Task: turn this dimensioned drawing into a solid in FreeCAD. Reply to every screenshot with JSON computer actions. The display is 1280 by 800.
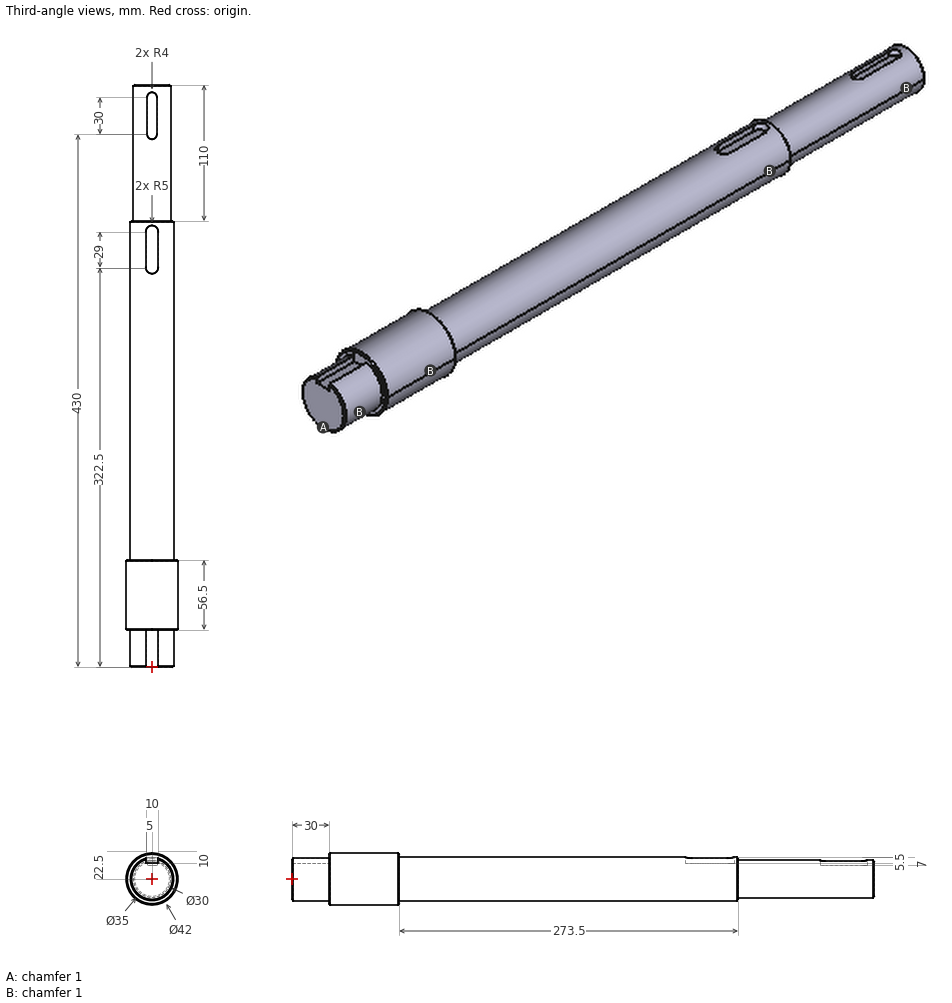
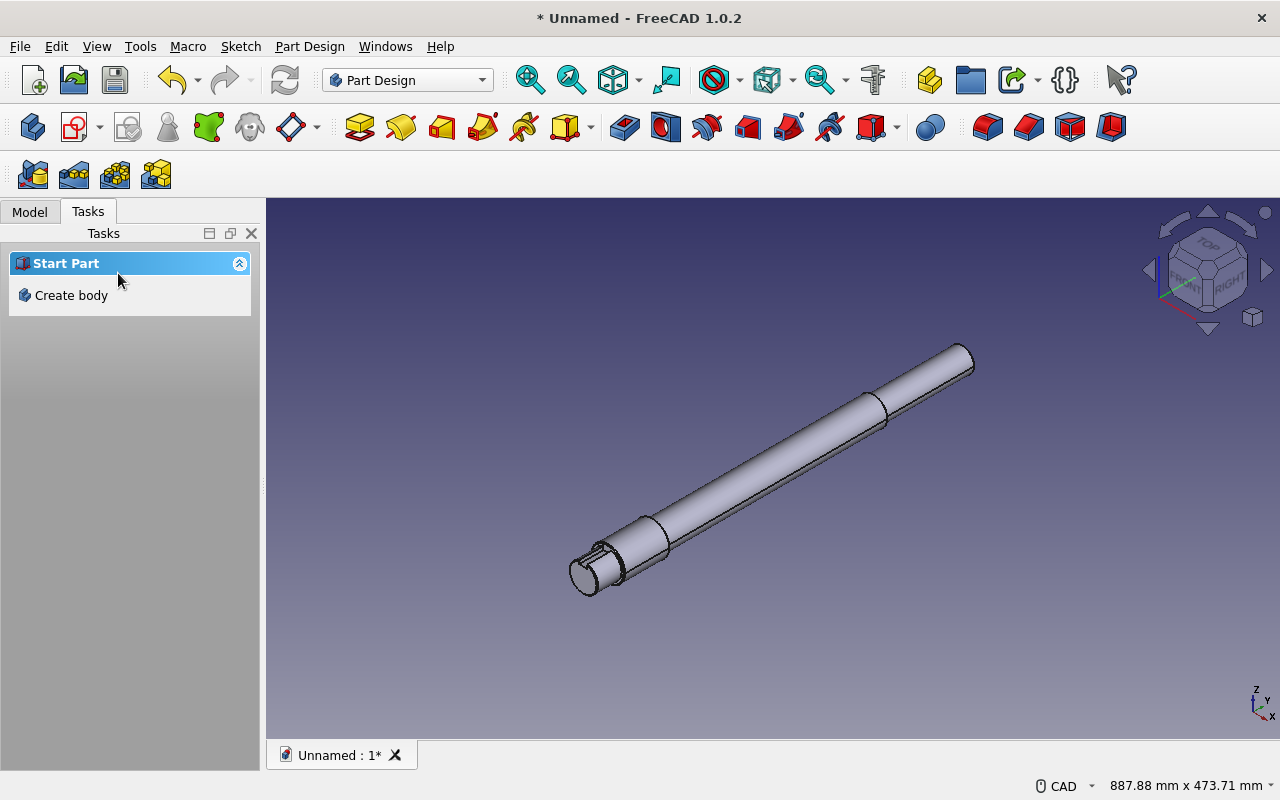
{"action": "left_click", "coordinate": [30, 212]}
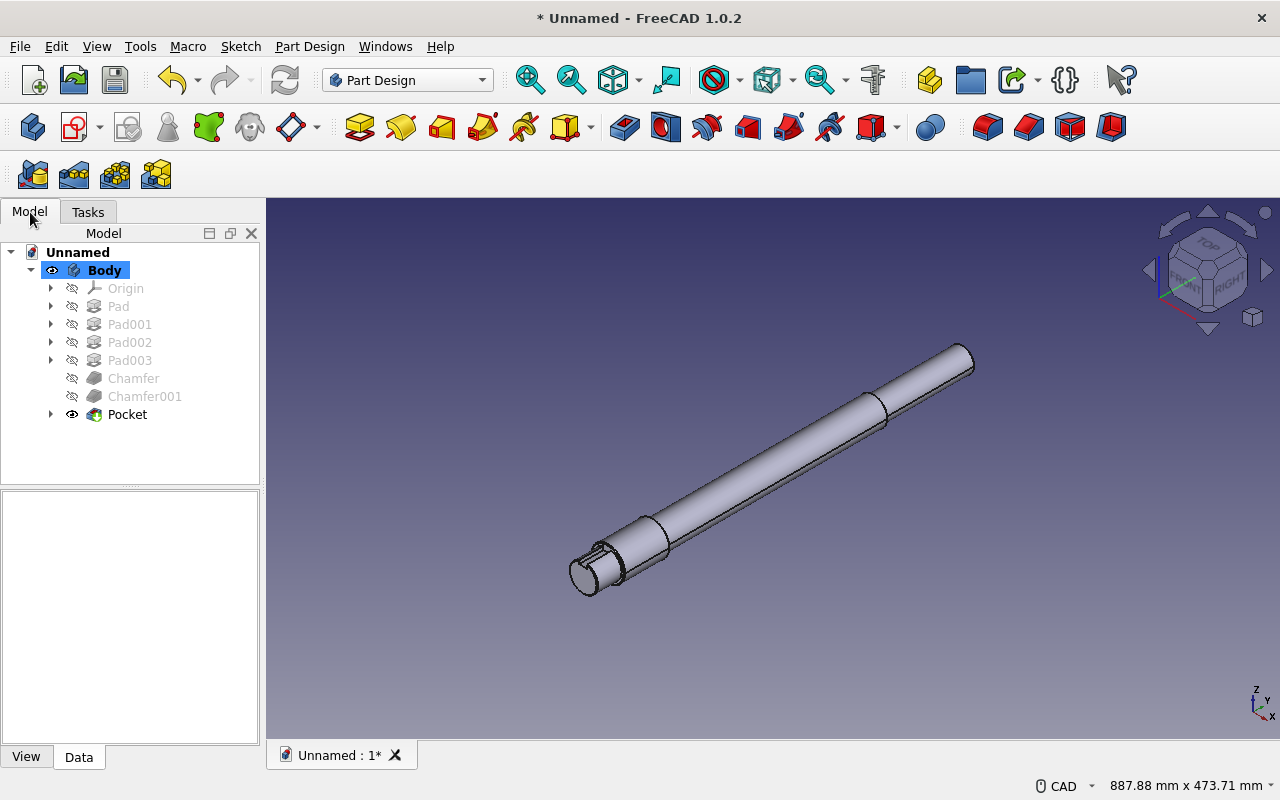
{"action": "left_click", "coordinate": [51, 288]}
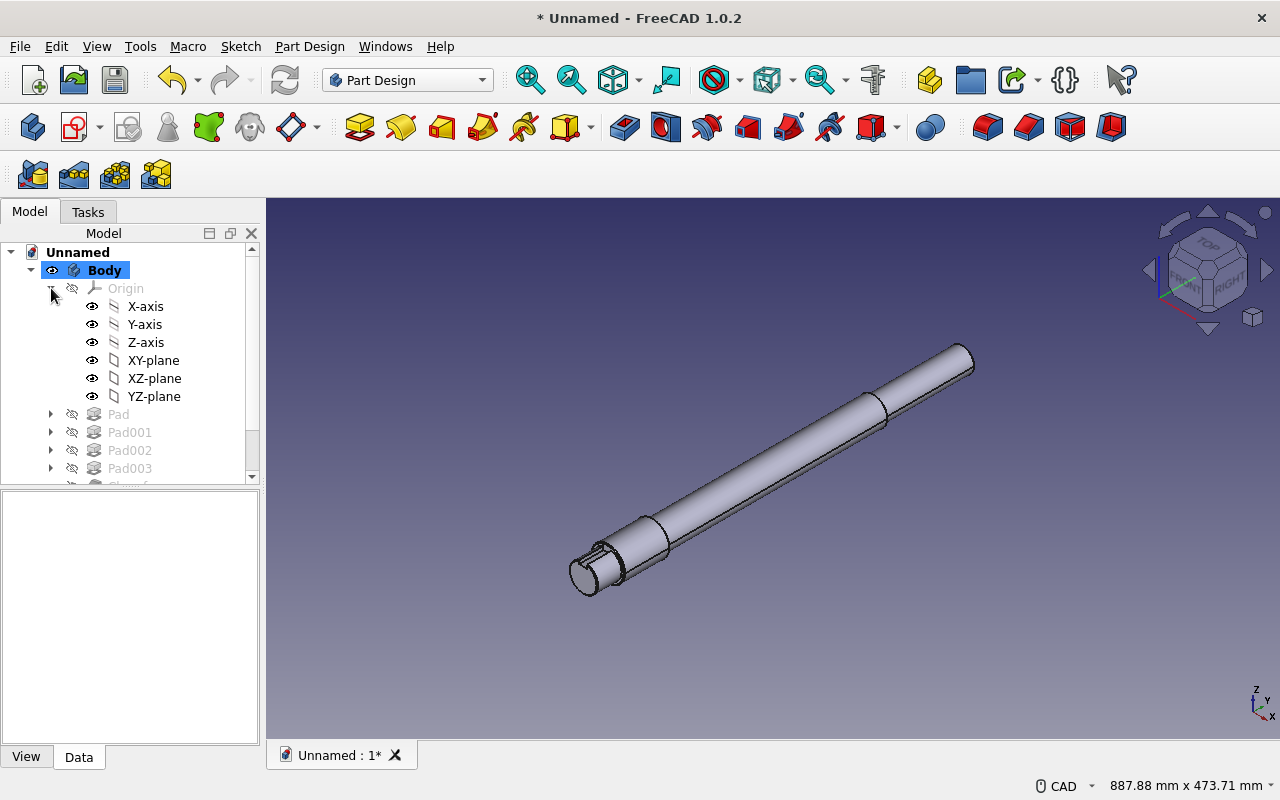
{"action": "left_click", "coordinate": [137, 360]}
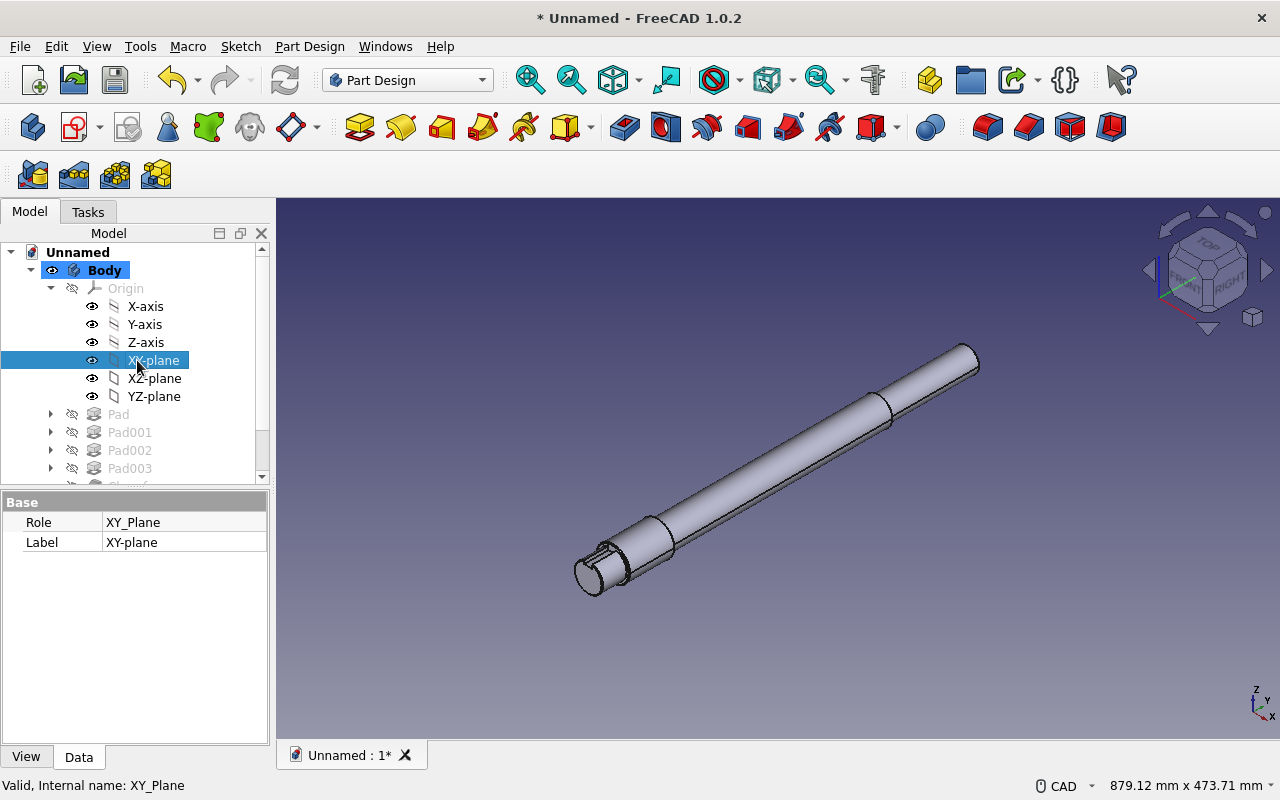
{"action": "left_click", "coordinate": [290, 128]}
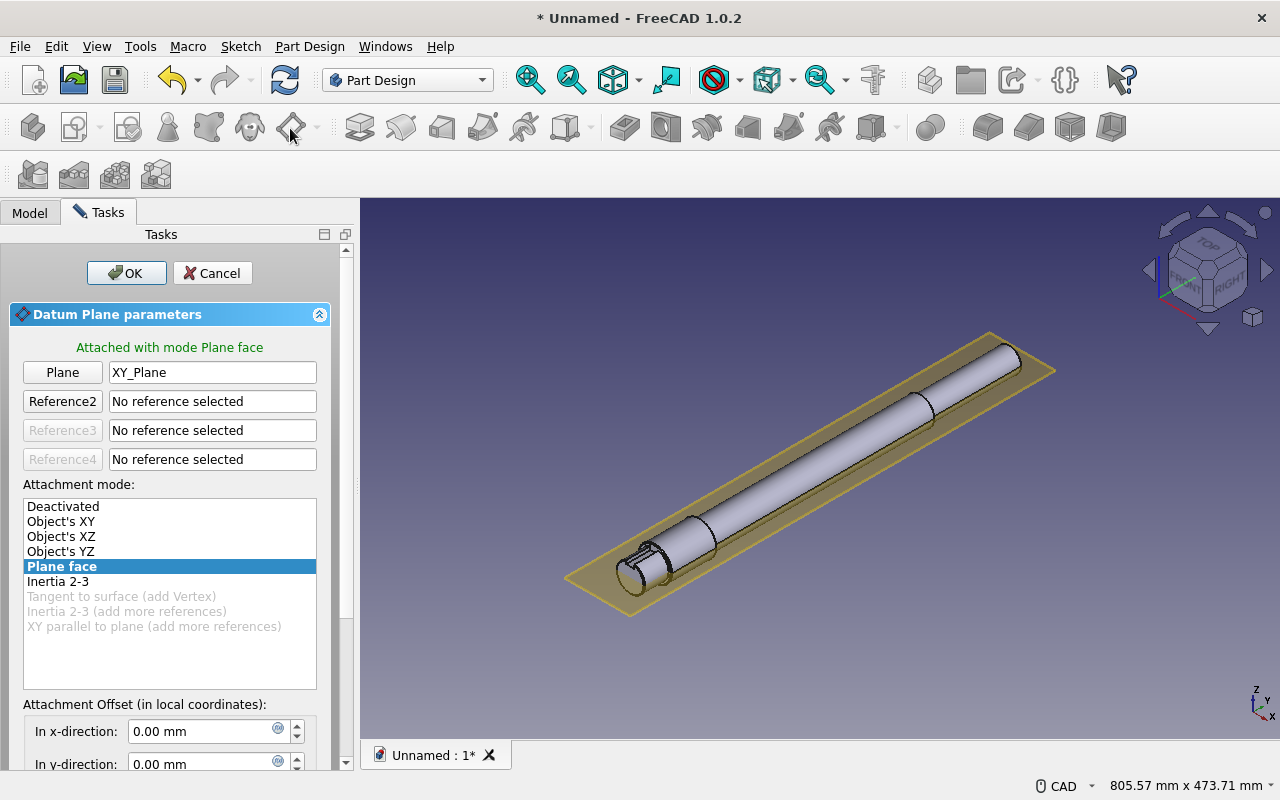
{"action": "scroll", "coordinate": [346, 507], "scroll_direction": "down", "scroll_amount": 2}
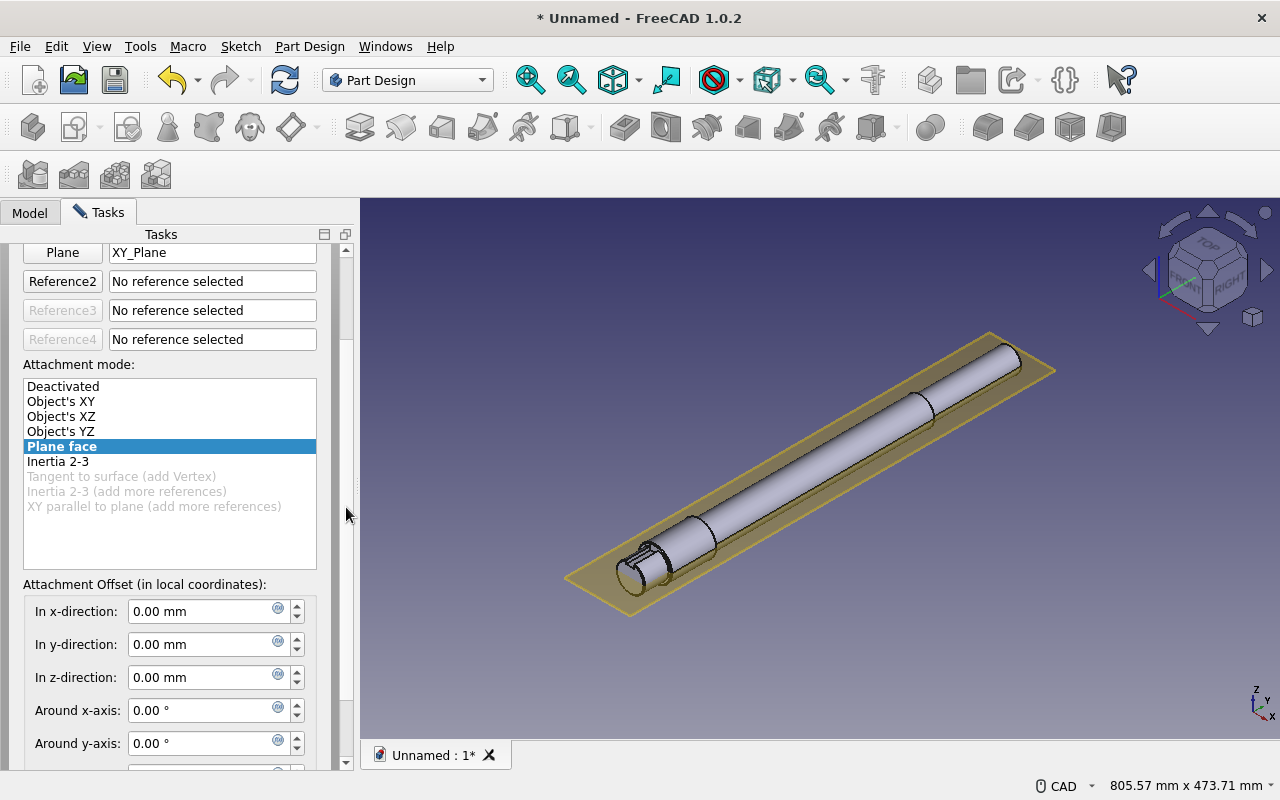
{"action": "triple_click", "coordinate": [210, 678]}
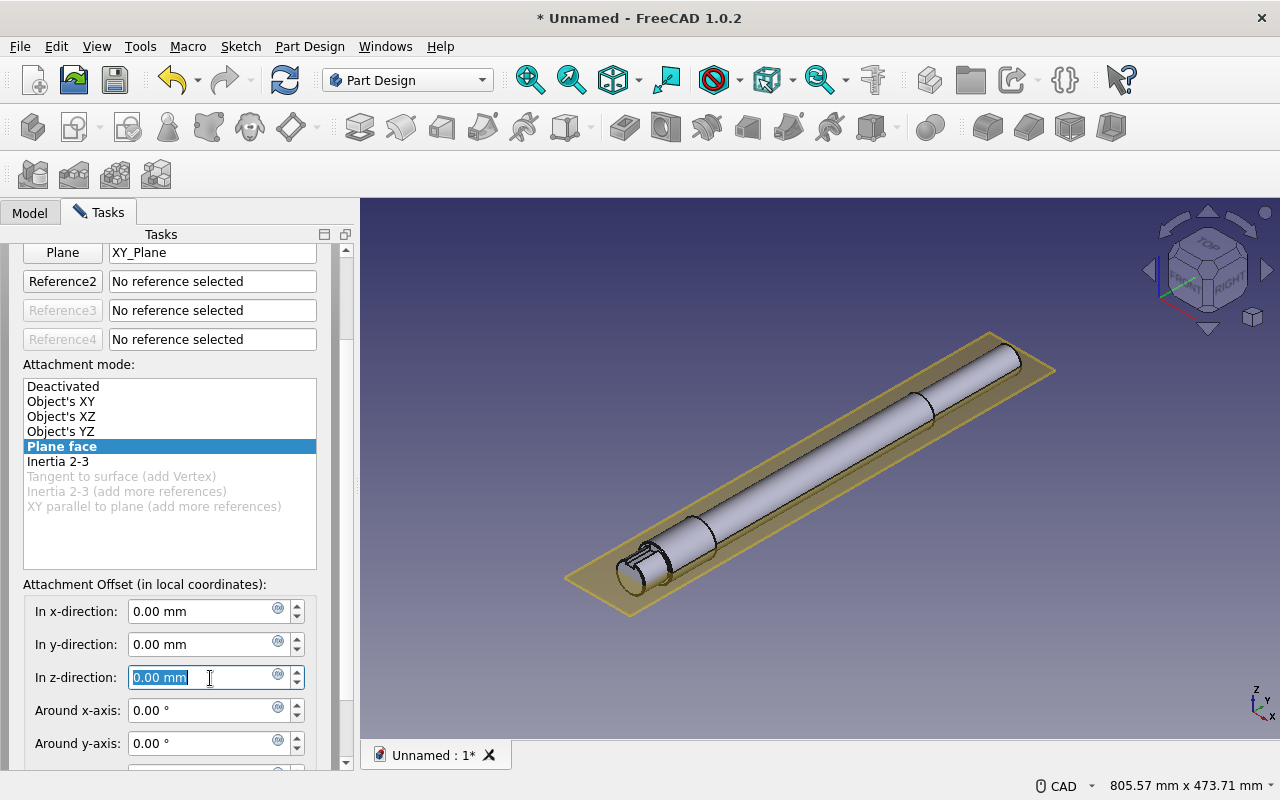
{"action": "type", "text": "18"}
{"action": "key", "text": "Tab"}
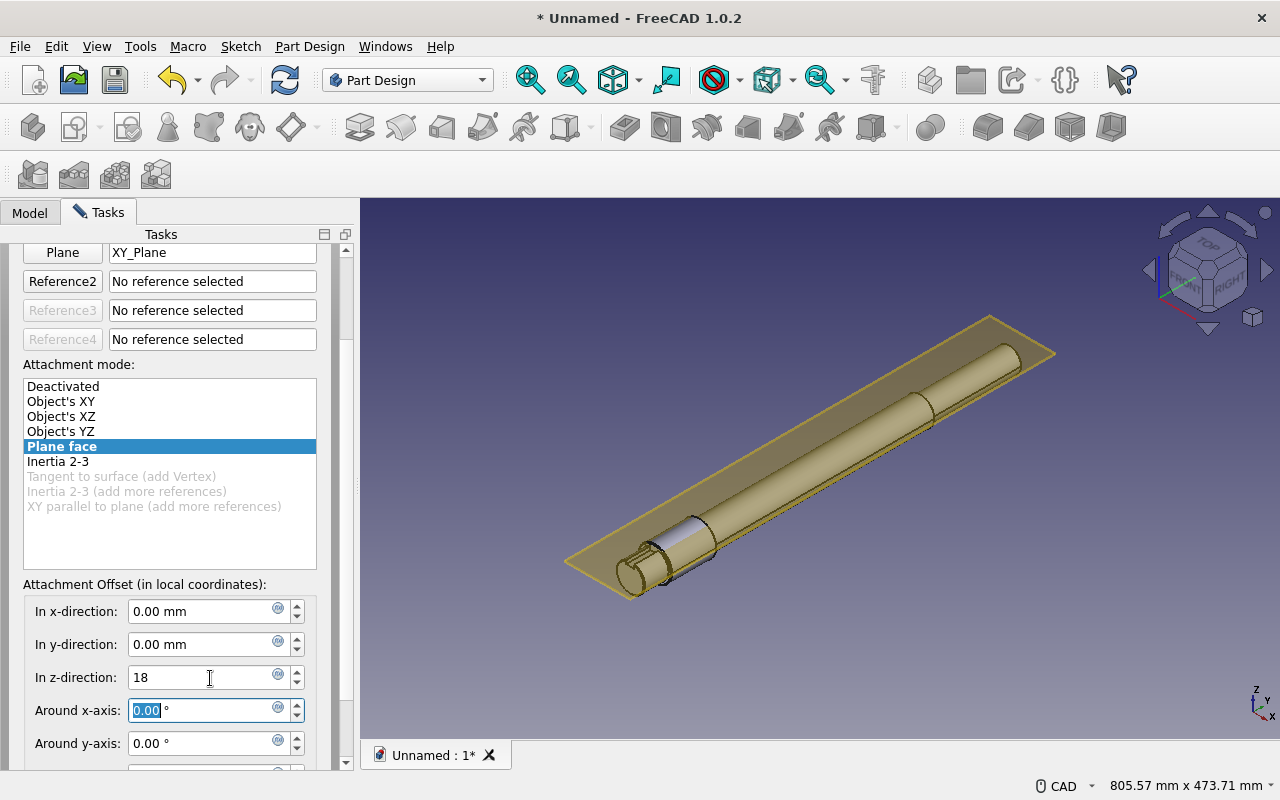
{"action": "scroll", "coordinate": [346, 507], "scroll_direction": "up", "scroll_amount": 3}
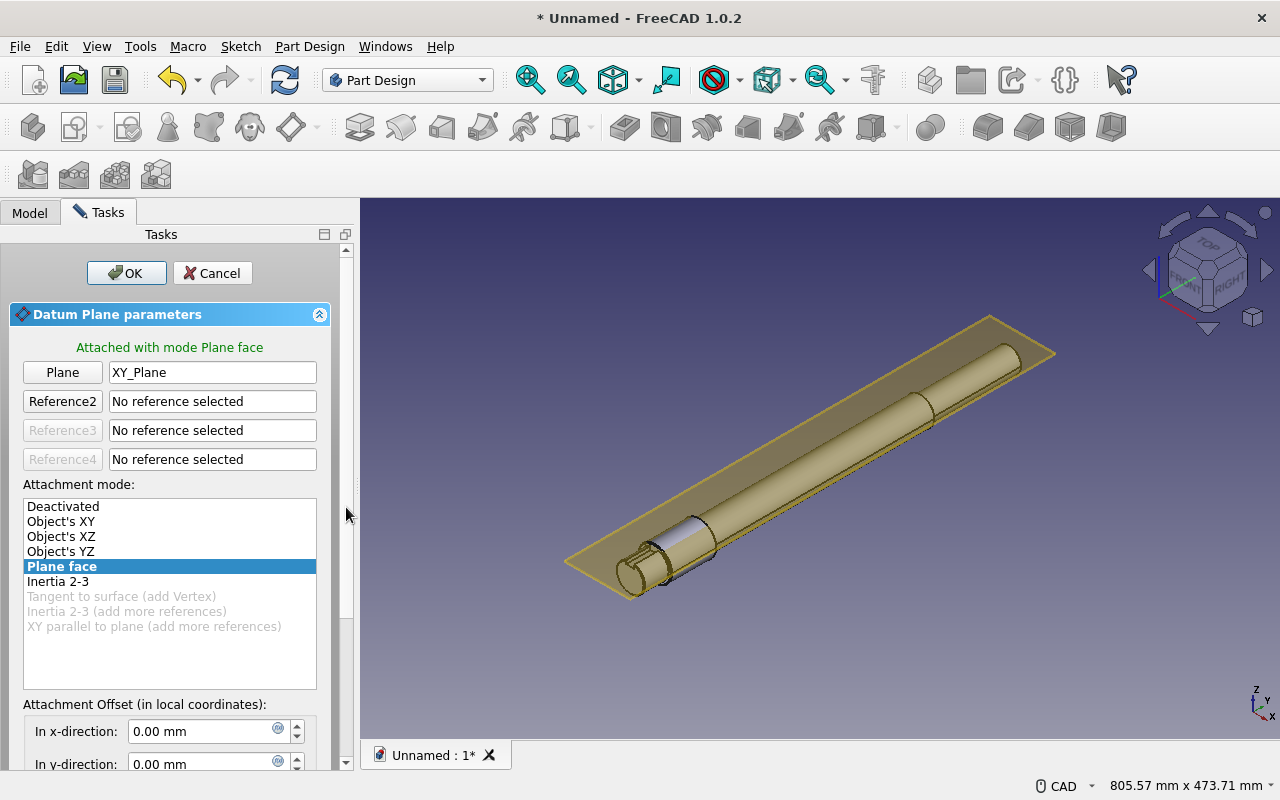
{"action": "left_click", "coordinate": [127, 273]}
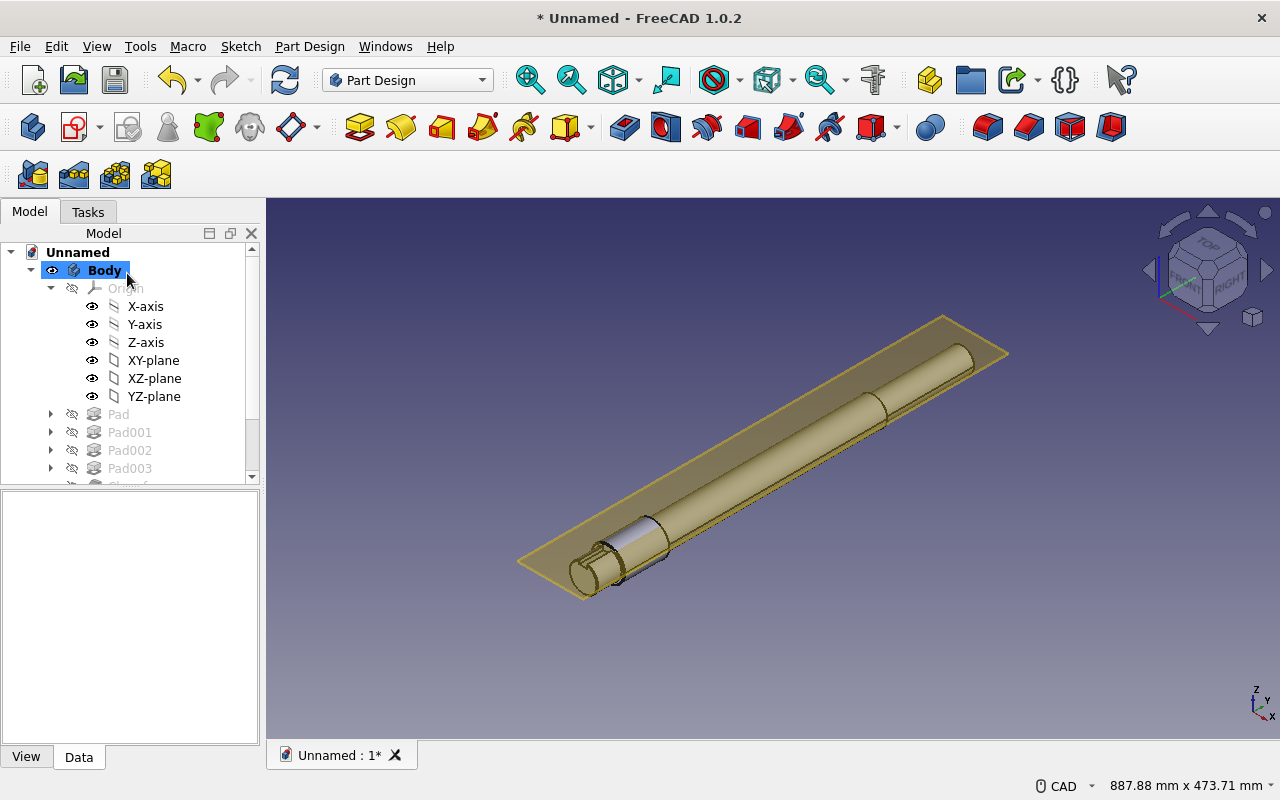
{"action": "scroll", "coordinate": [101, 356], "scroll_direction": "down", "scroll_amount": 3}